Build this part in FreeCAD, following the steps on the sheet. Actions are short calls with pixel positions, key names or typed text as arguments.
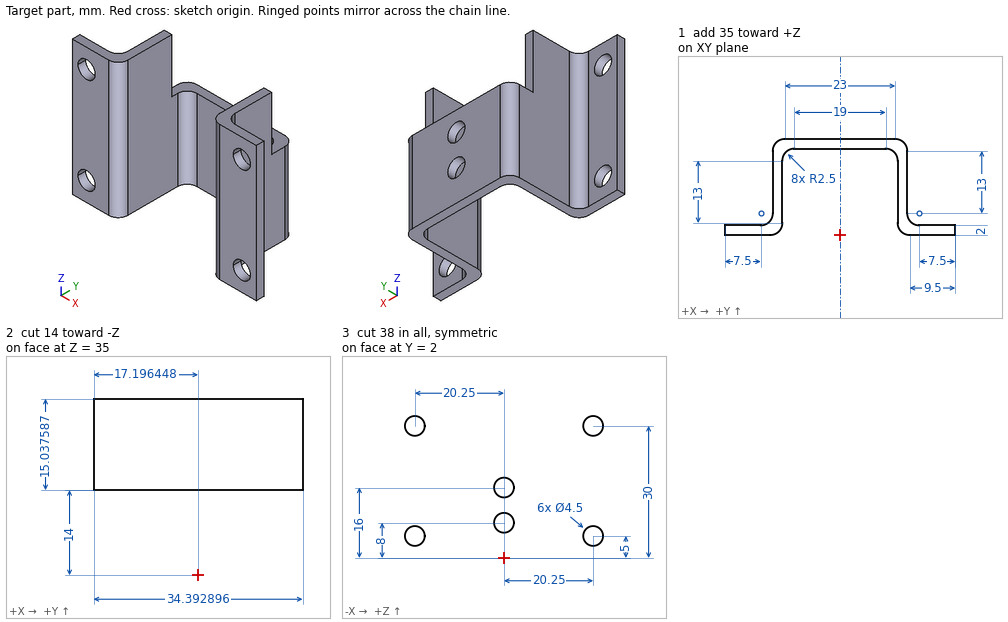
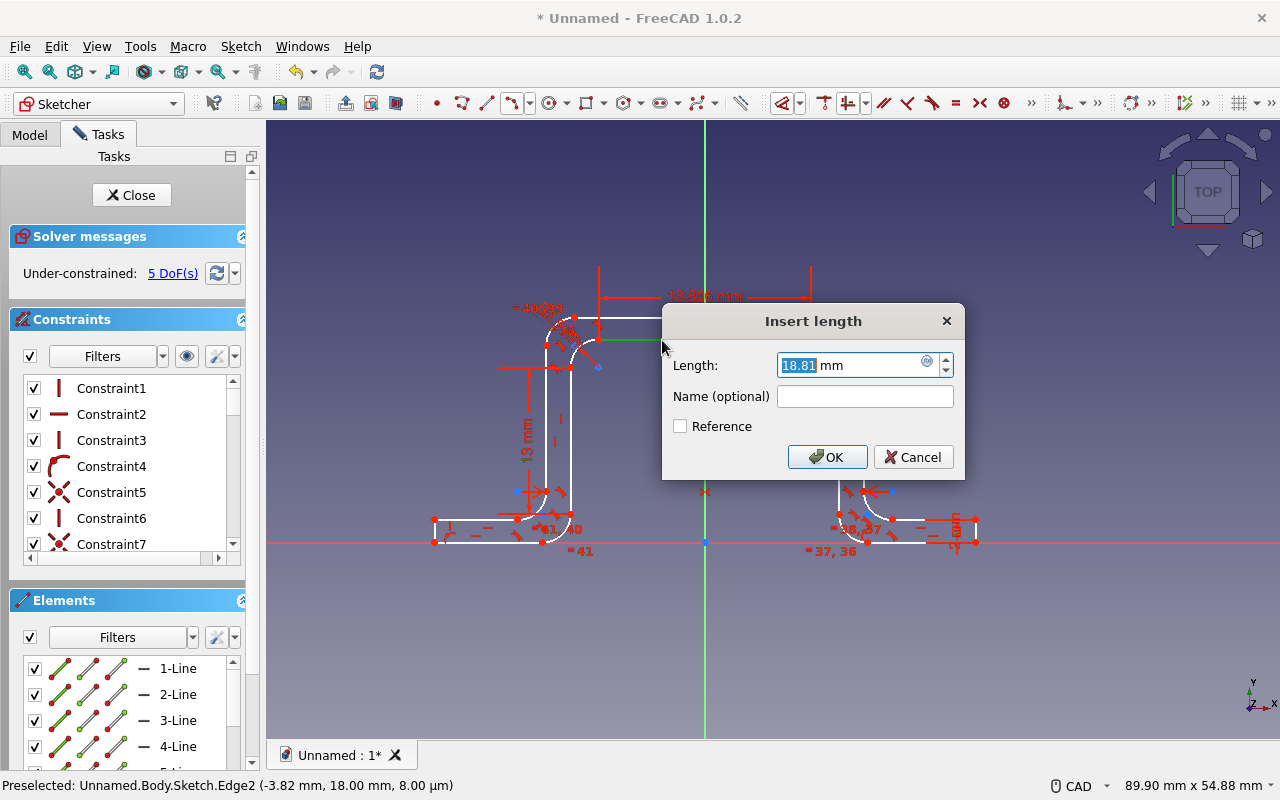
text(19)
key(Return)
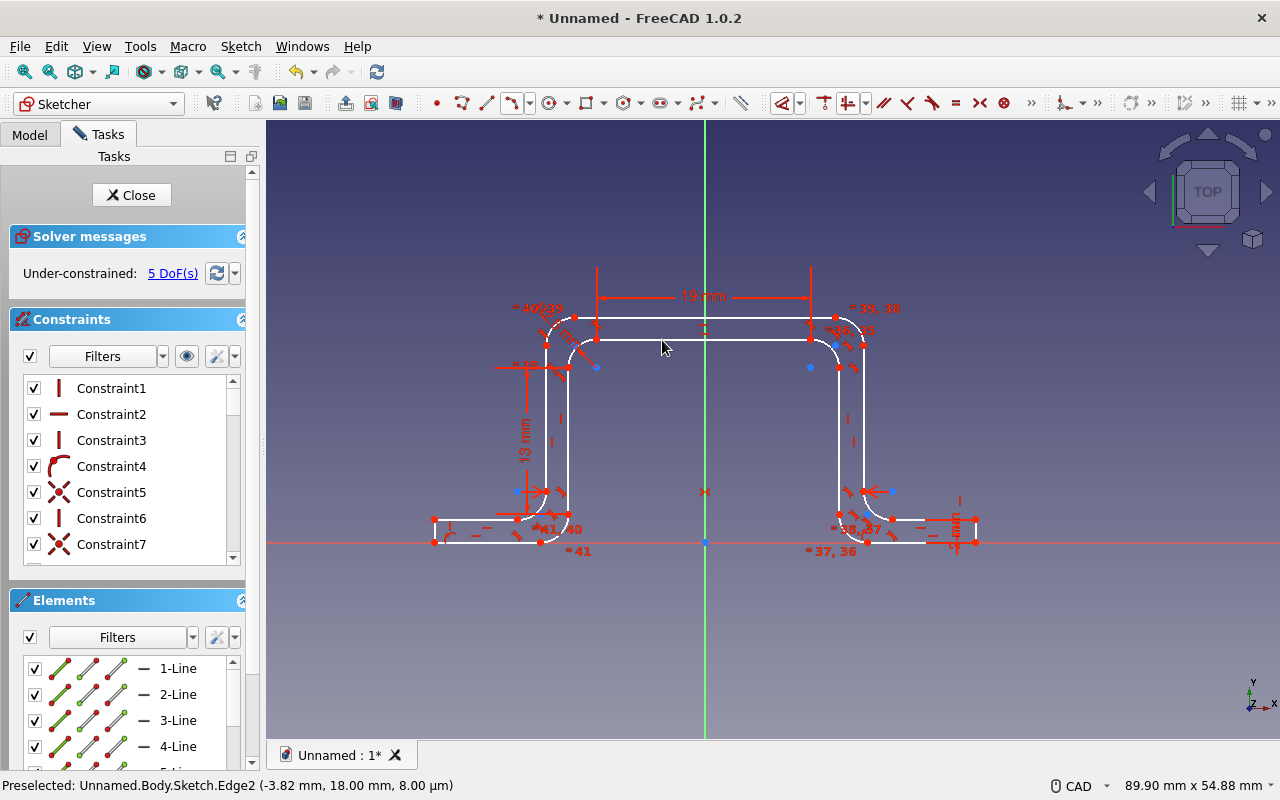
click(864, 448)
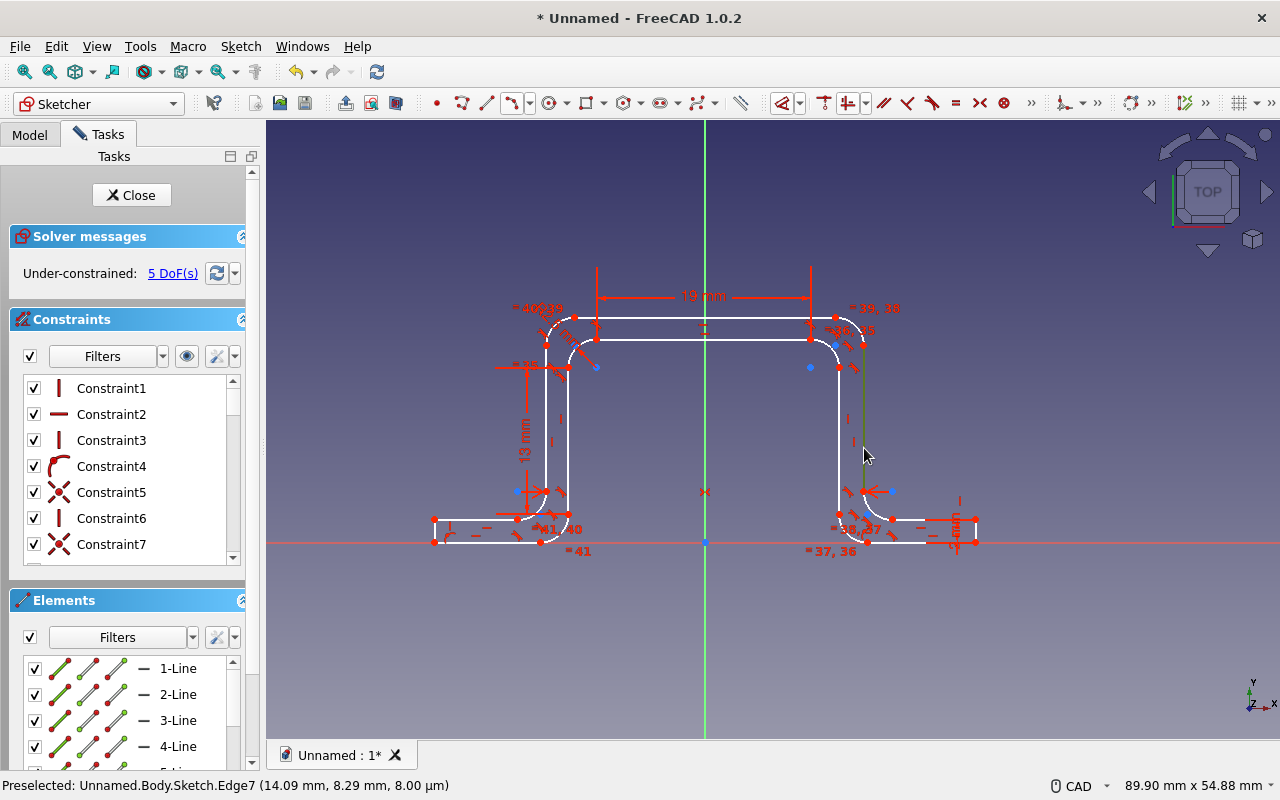
key(i)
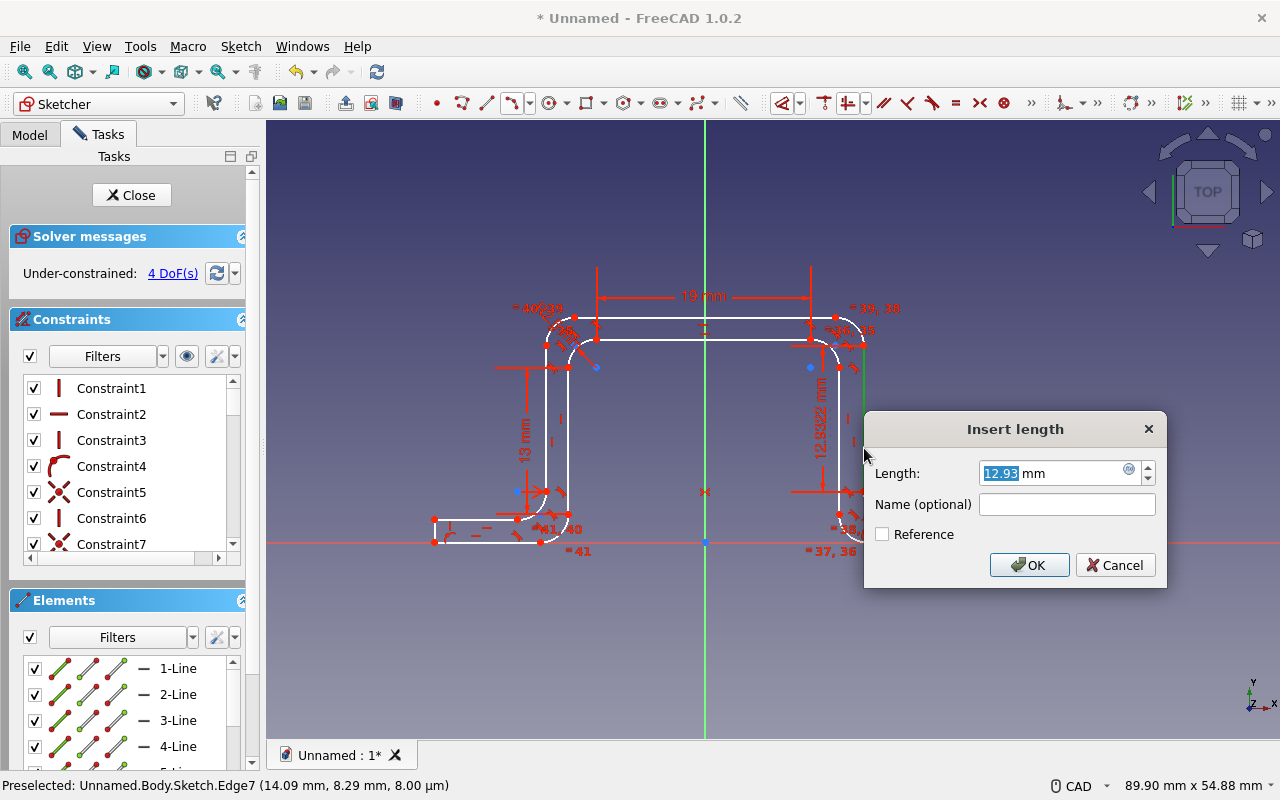
text(13)
key(Return)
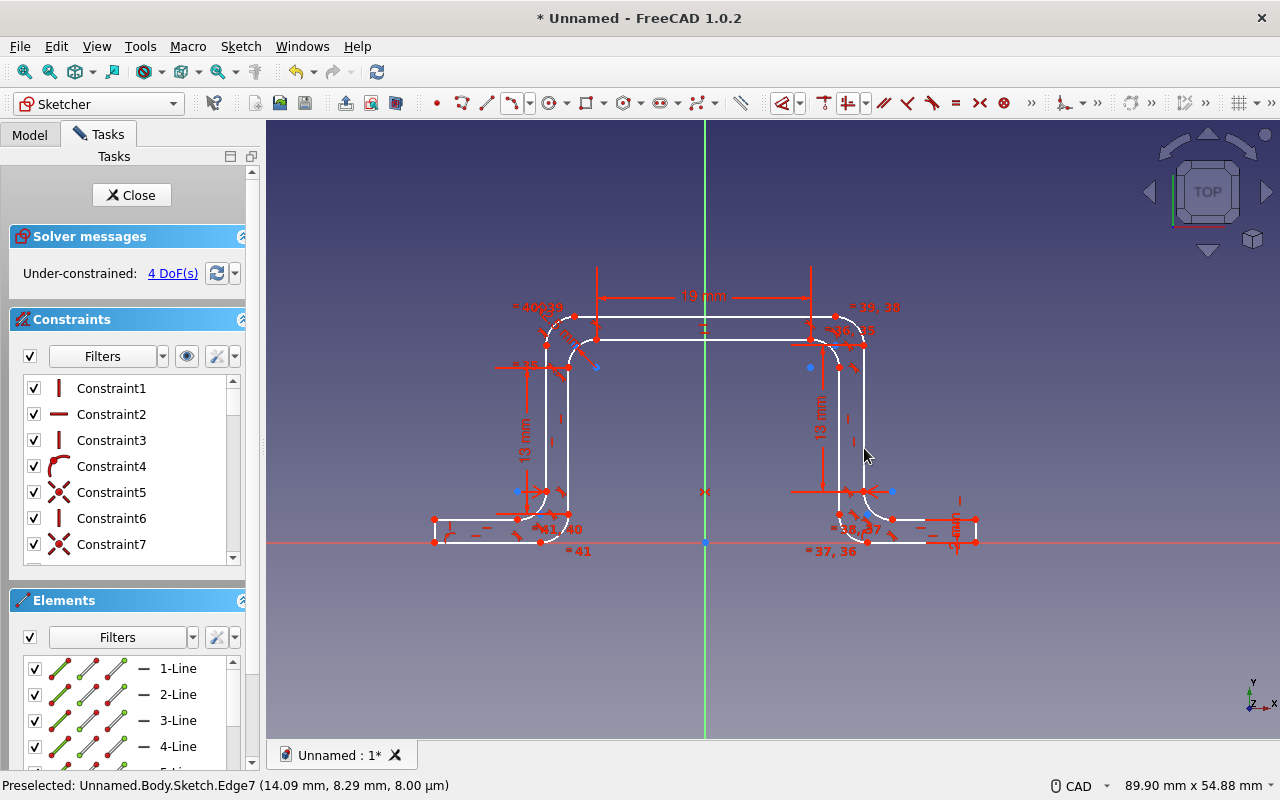
click(757, 317)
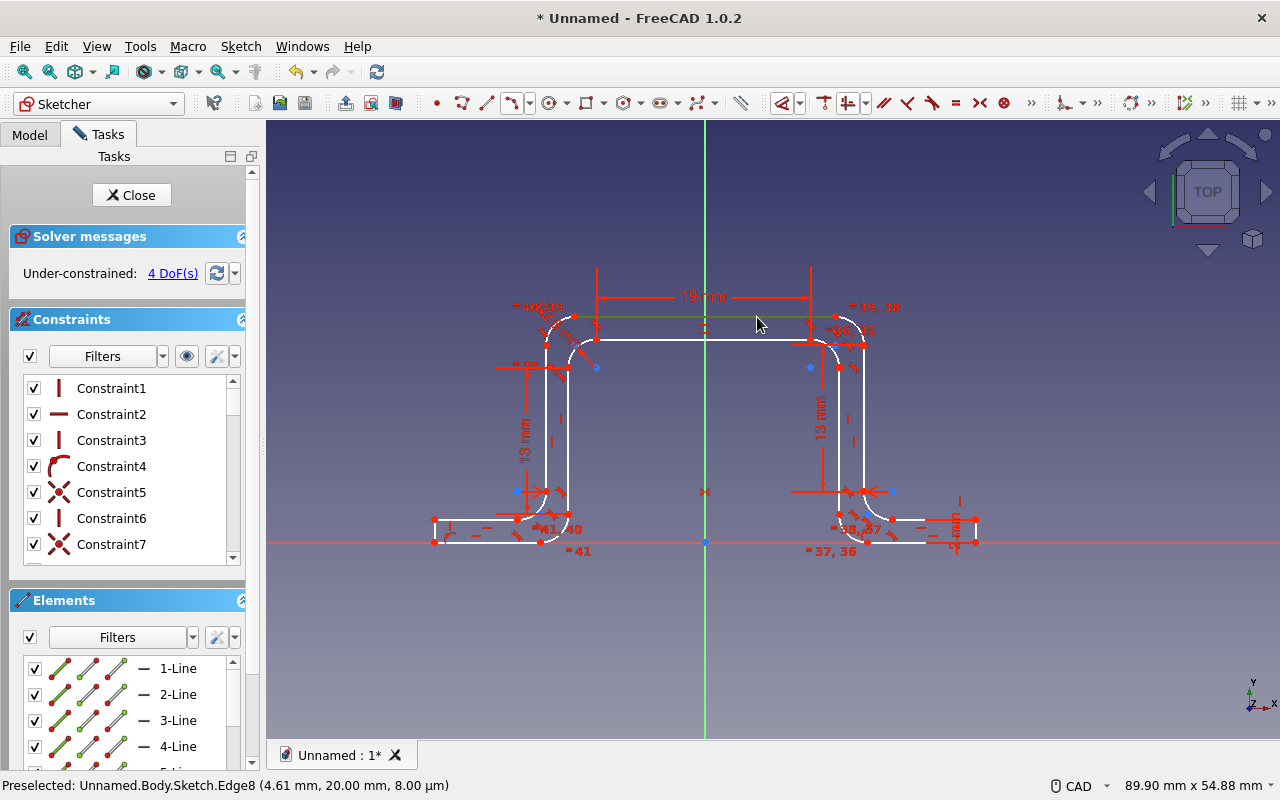
click(800, 104)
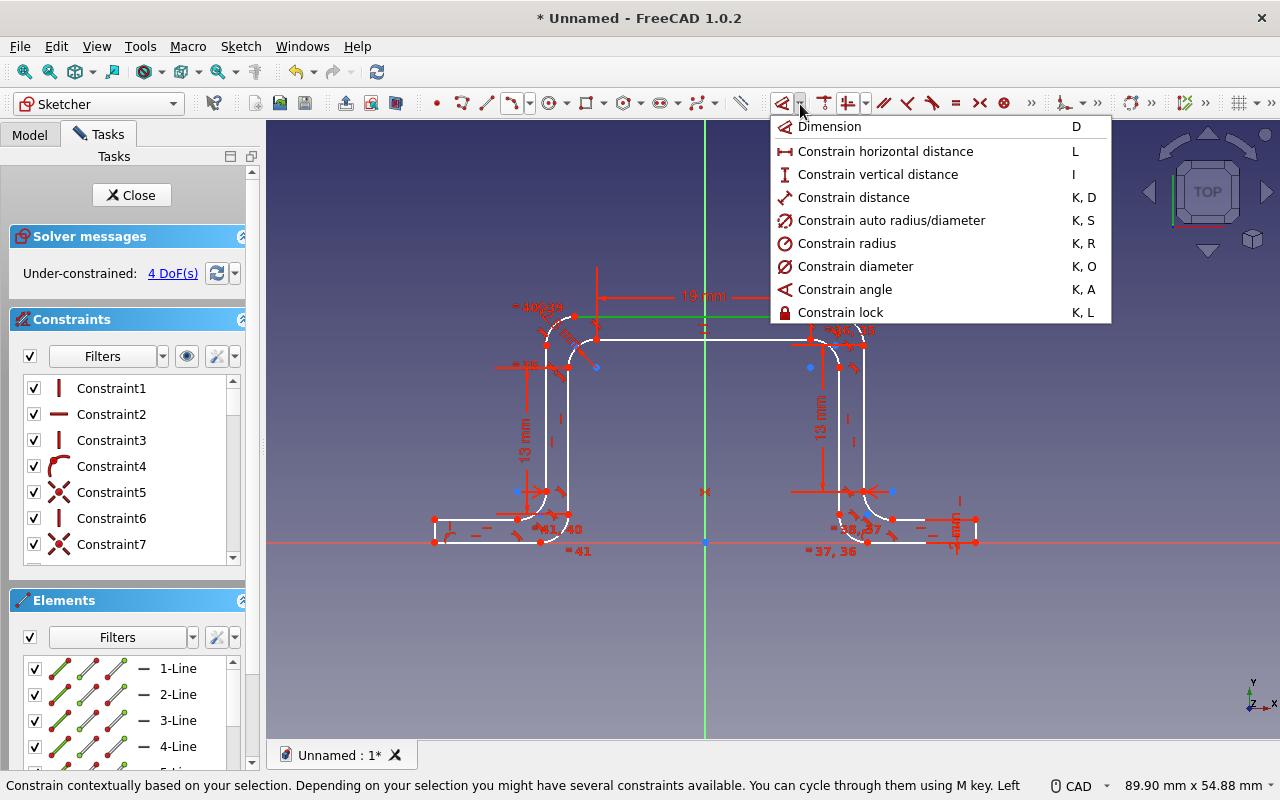
click(941, 152)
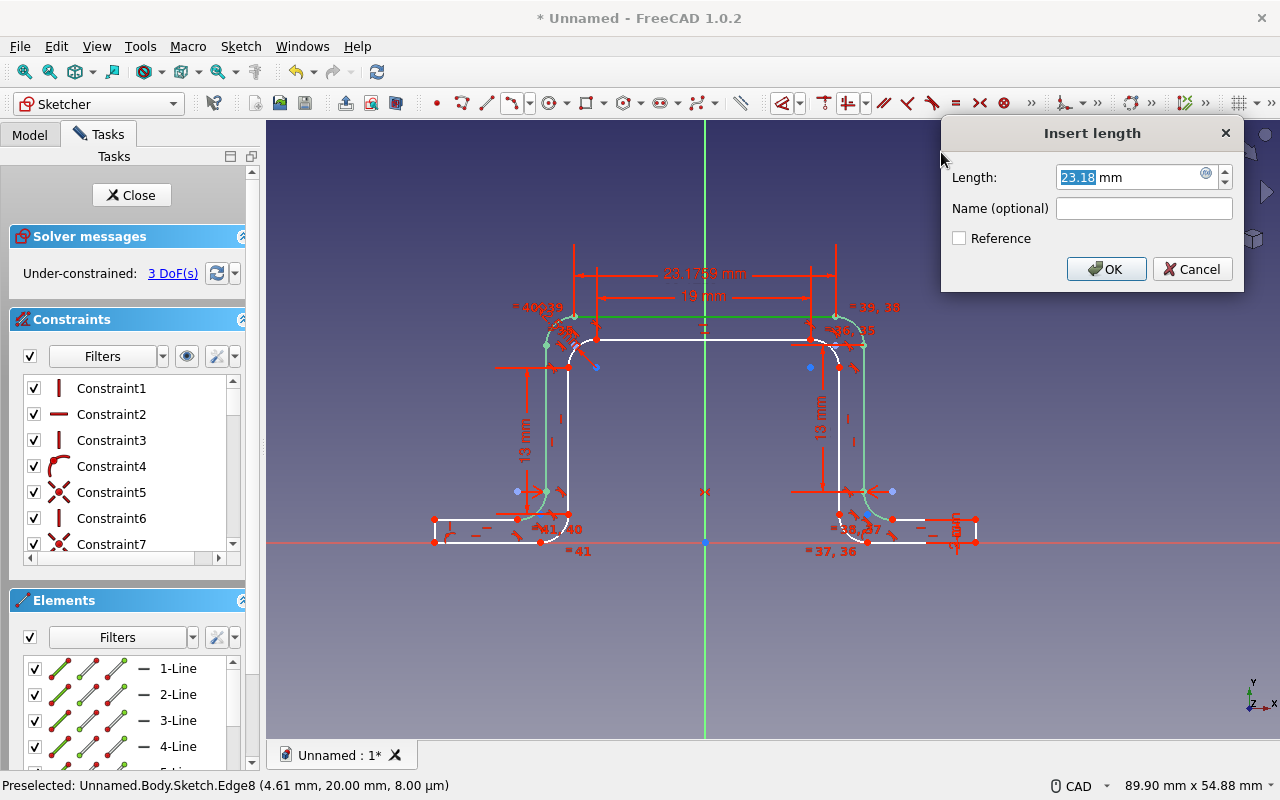
text(23)
key(Return)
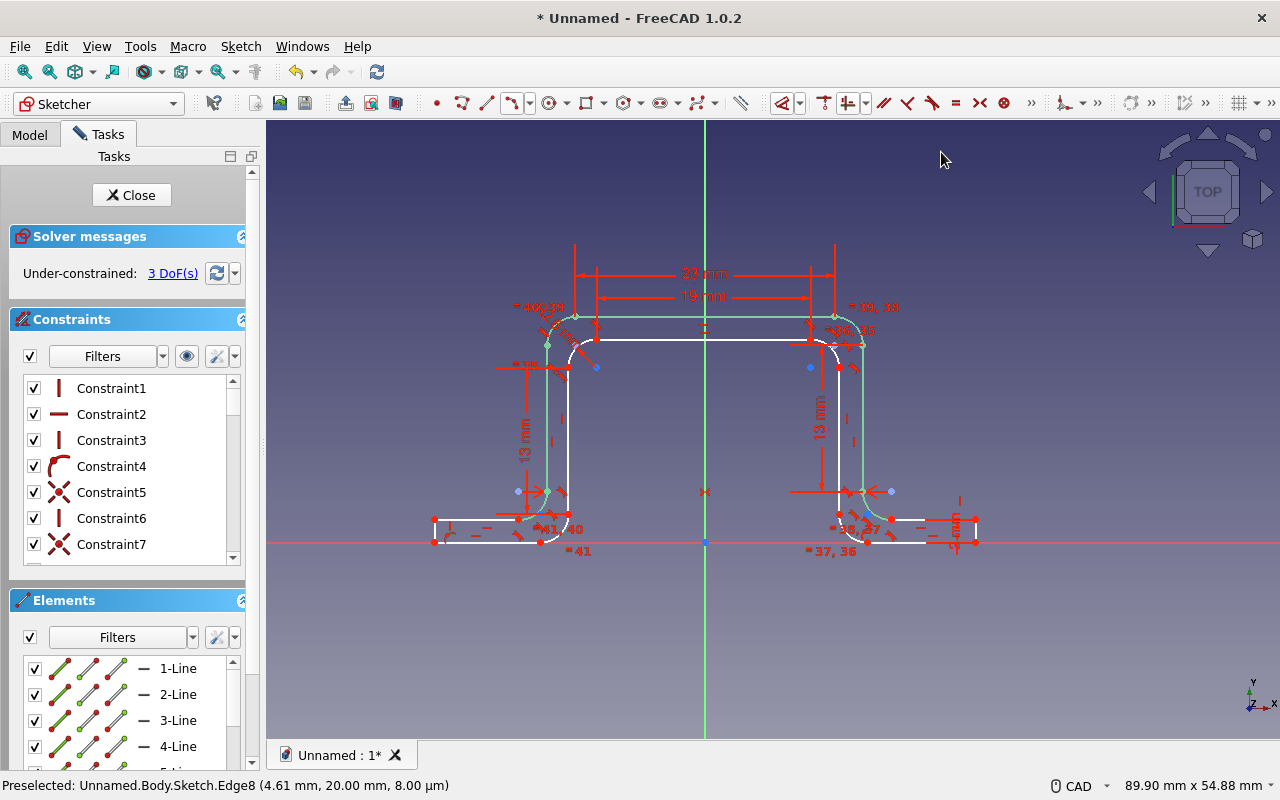
click(900, 543)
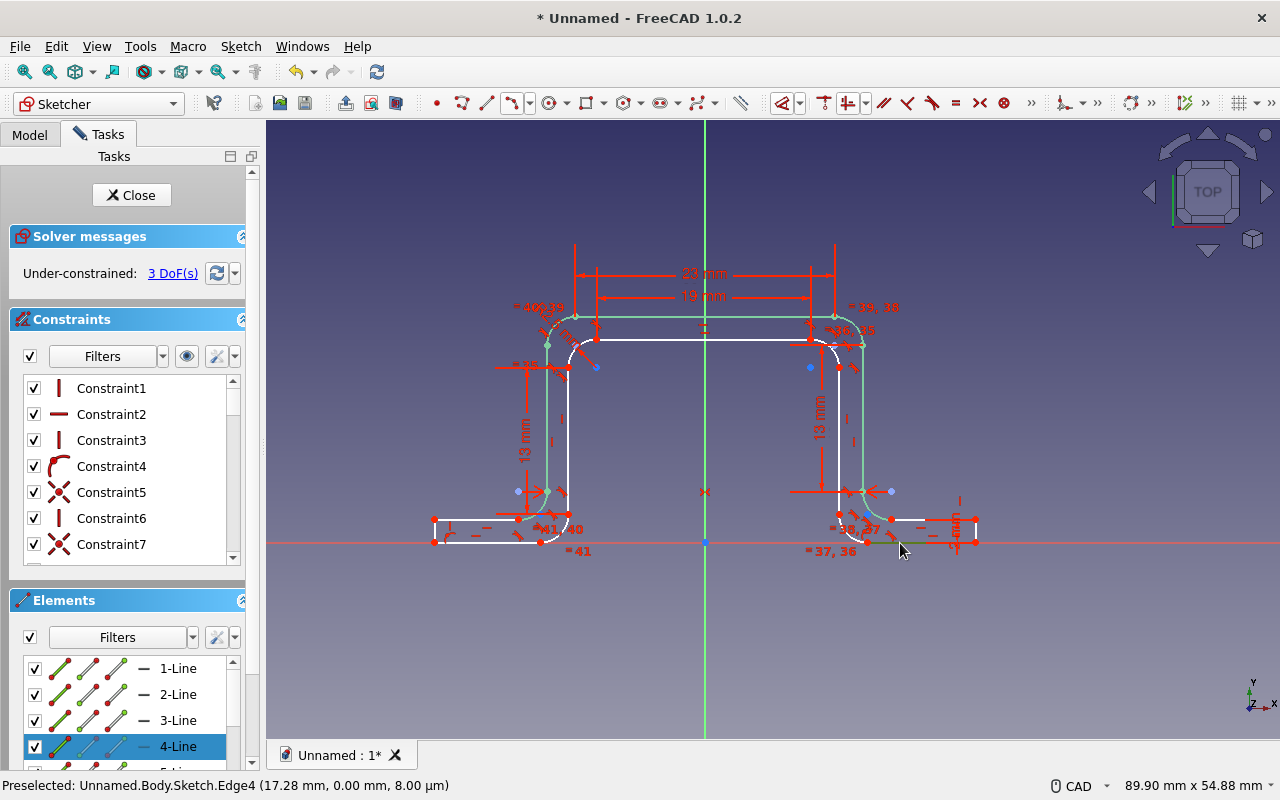
click(800, 104)